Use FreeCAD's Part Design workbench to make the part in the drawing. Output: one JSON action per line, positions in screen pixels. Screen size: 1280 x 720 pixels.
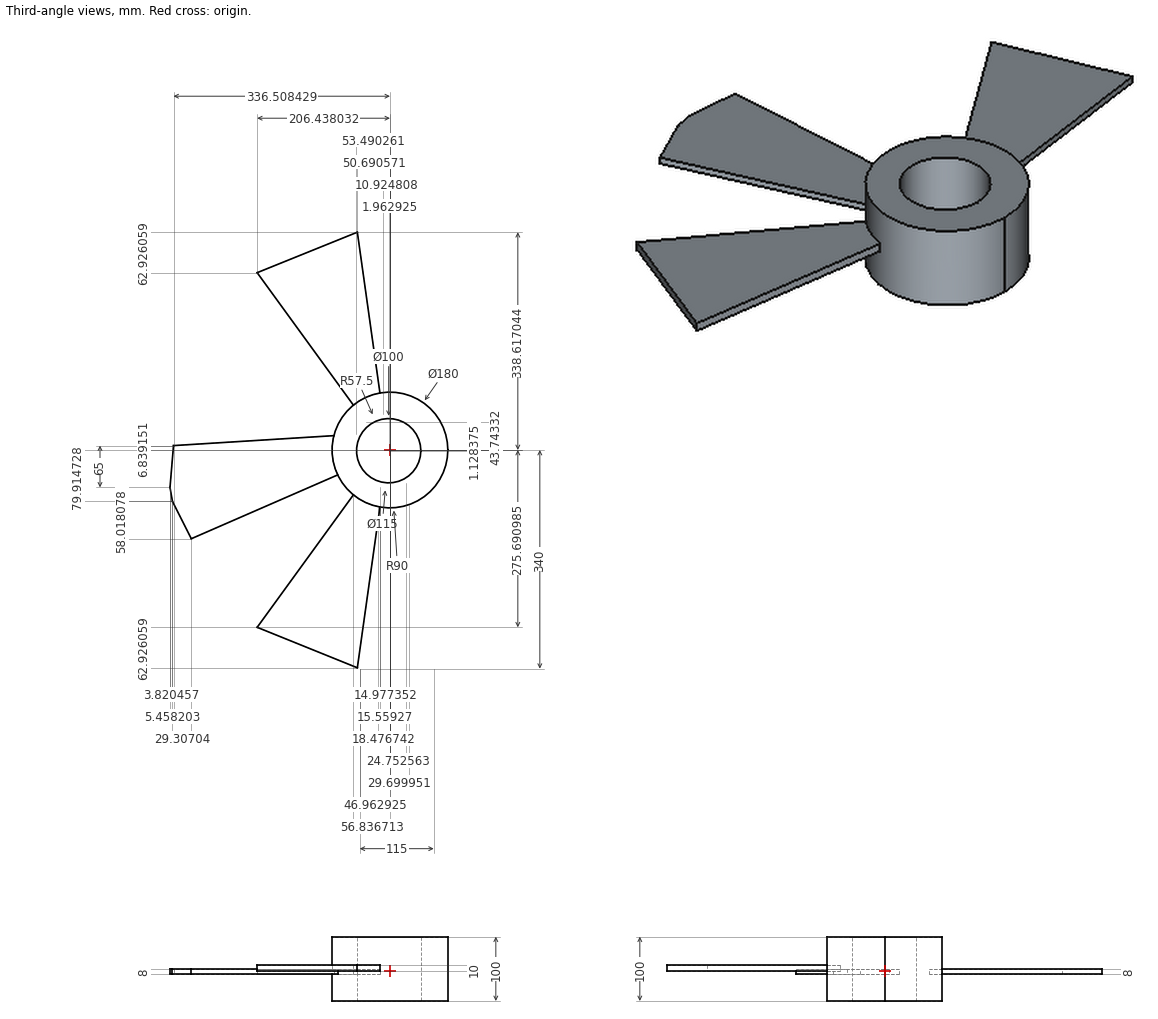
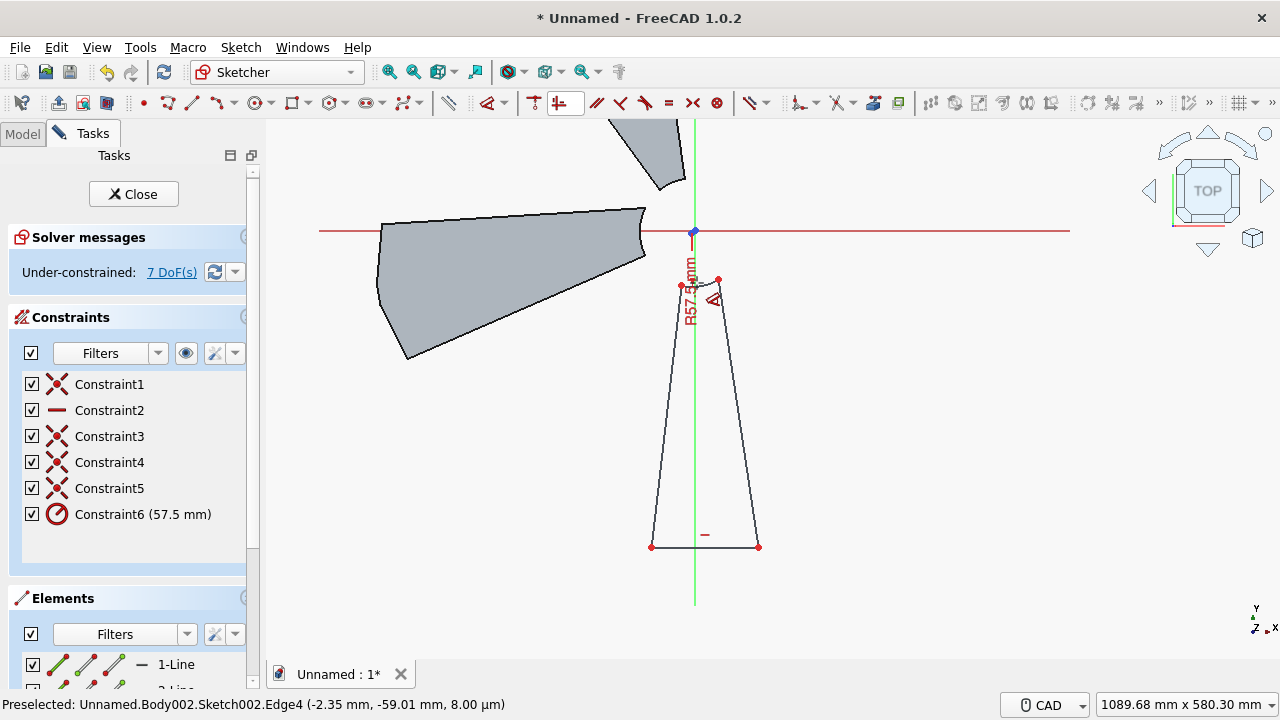
{"action": "left_click", "coordinate": [684, 548]}
{"action": "left_click", "coordinate": [680, 582]}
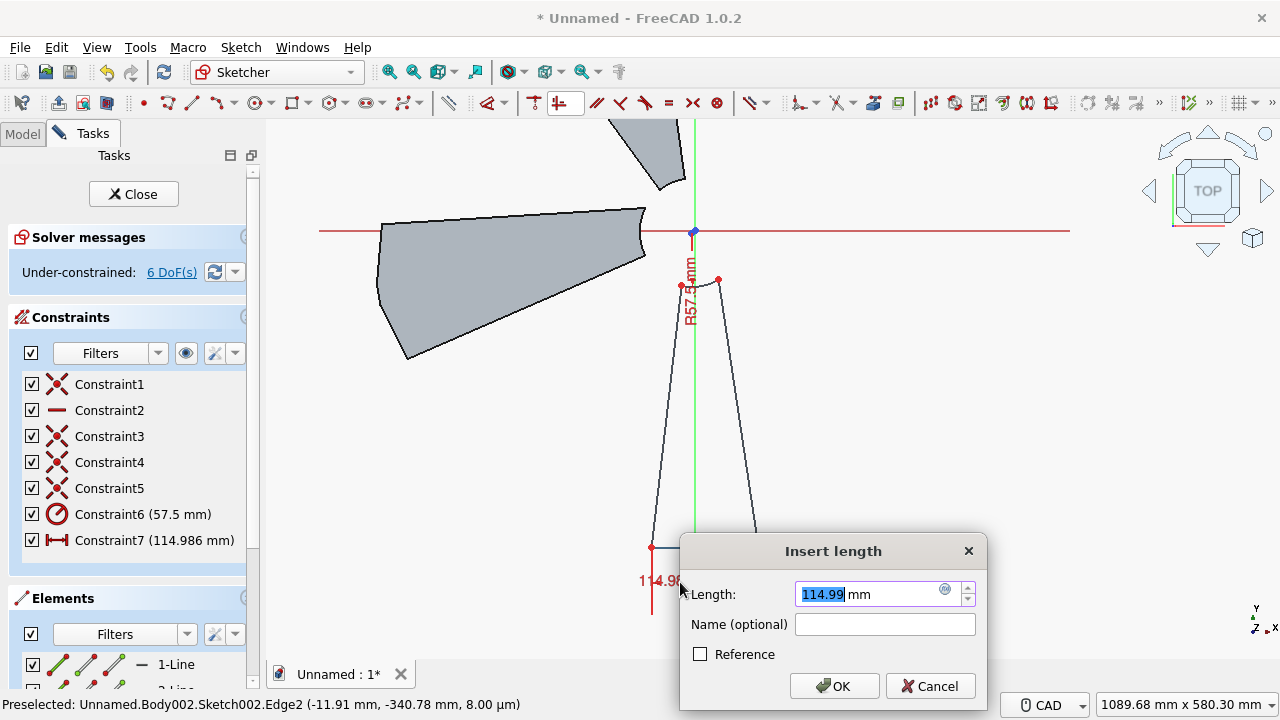
{"action": "type", "text": "115"}
{"action": "key", "text": "Return"}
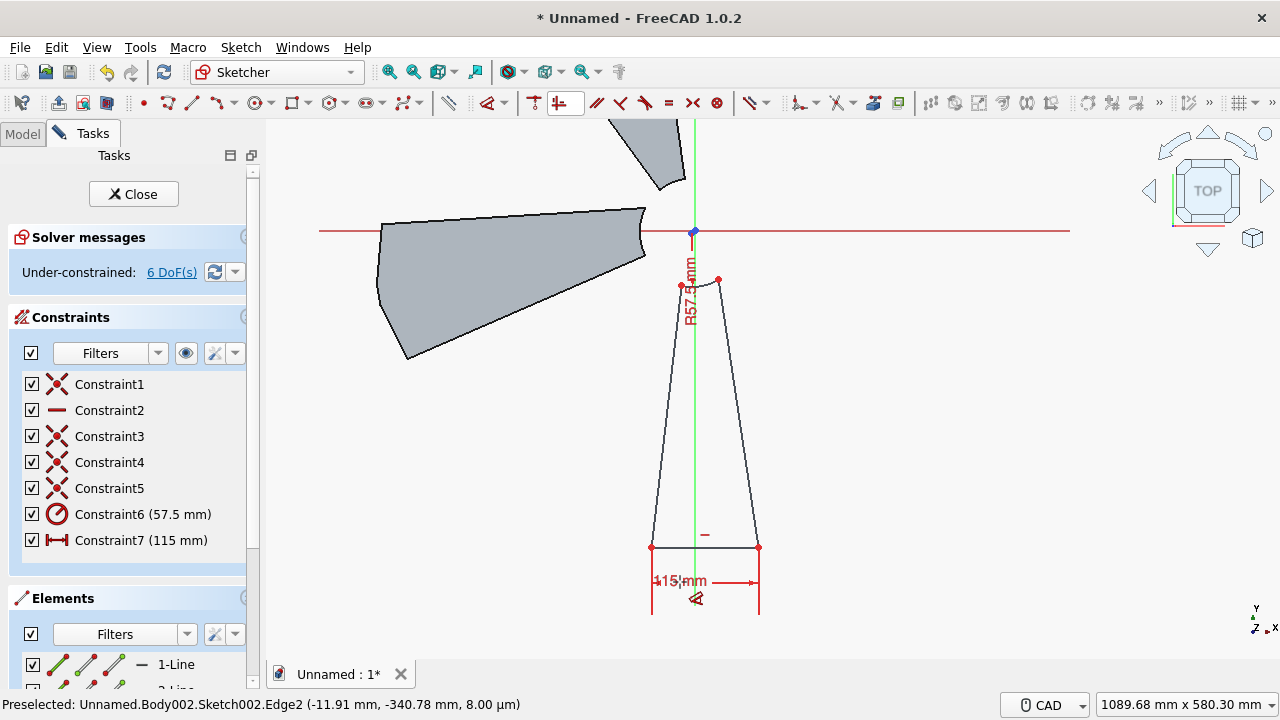
{"action": "left_click", "coordinate": [652, 548]}
{"action": "left_click", "coordinate": [618, 389]}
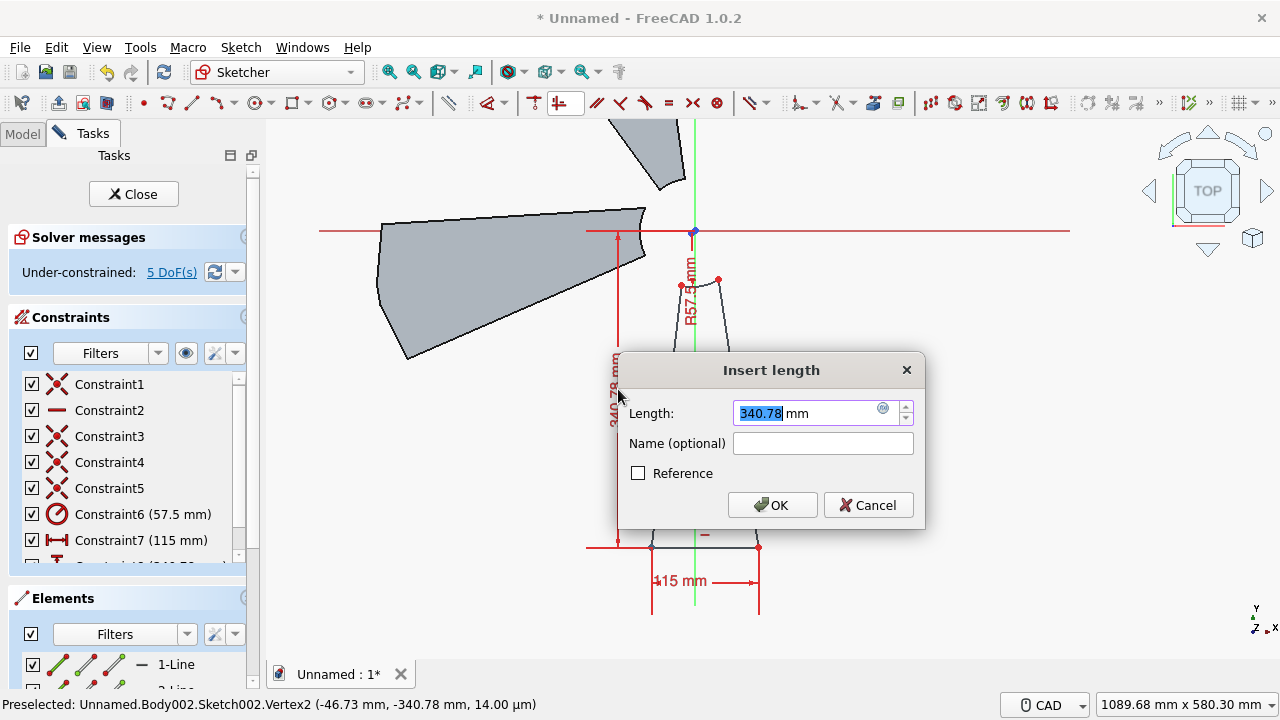
{"action": "type", "text": "340"}
{"action": "key", "text": "Return"}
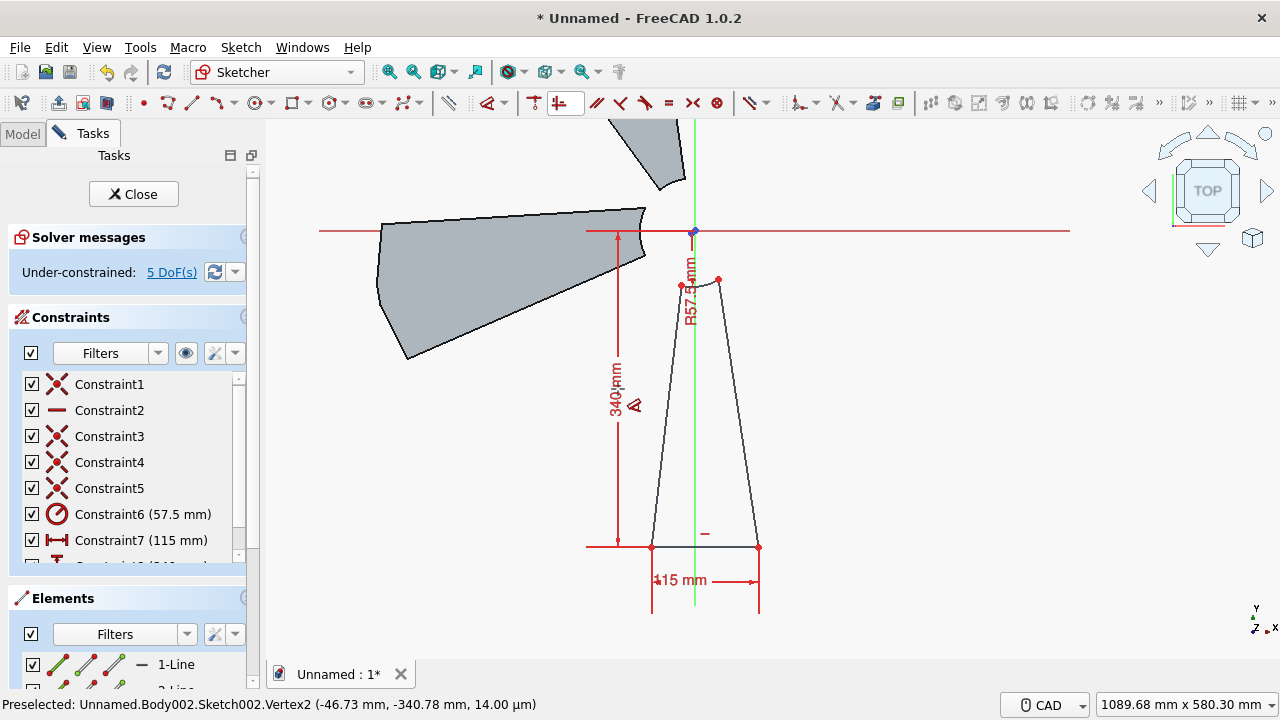
{"action": "scroll", "coordinate": [692, 233], "scroll_direction": "up", "scroll_amount": 16}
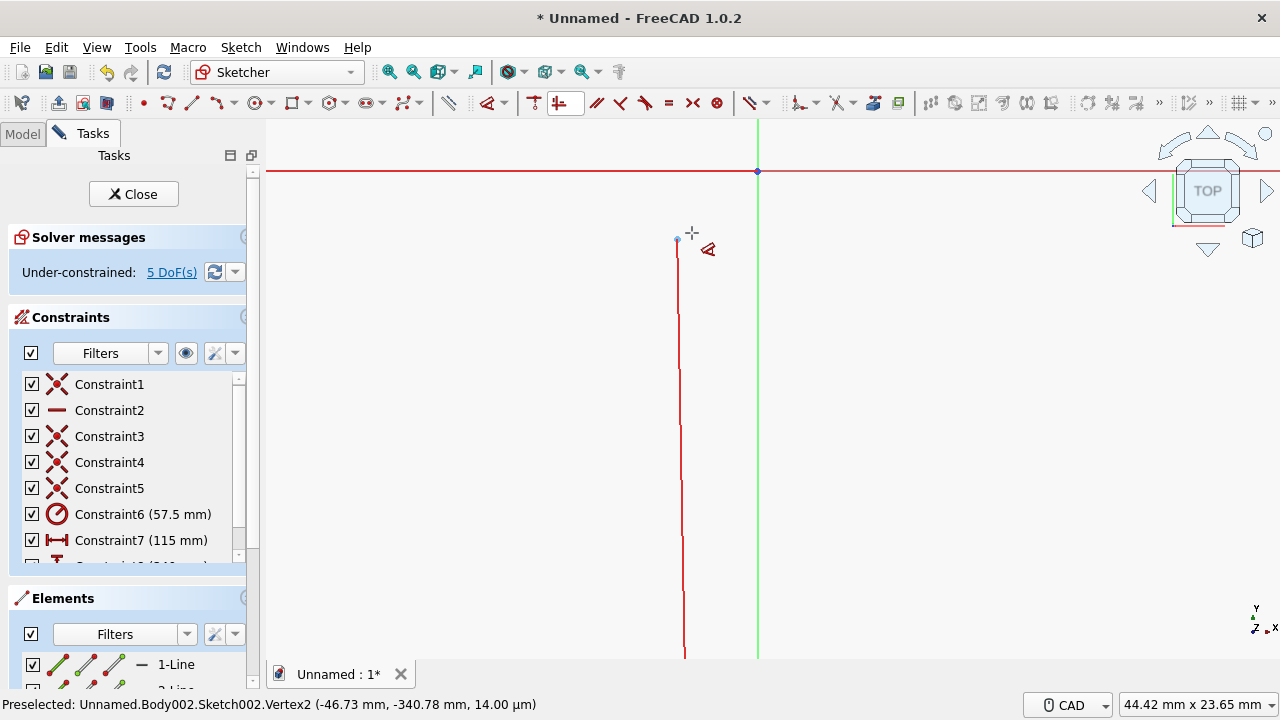
{"action": "left_click", "coordinate": [677, 239]}
{"action": "left_click", "coordinate": [717, 273]}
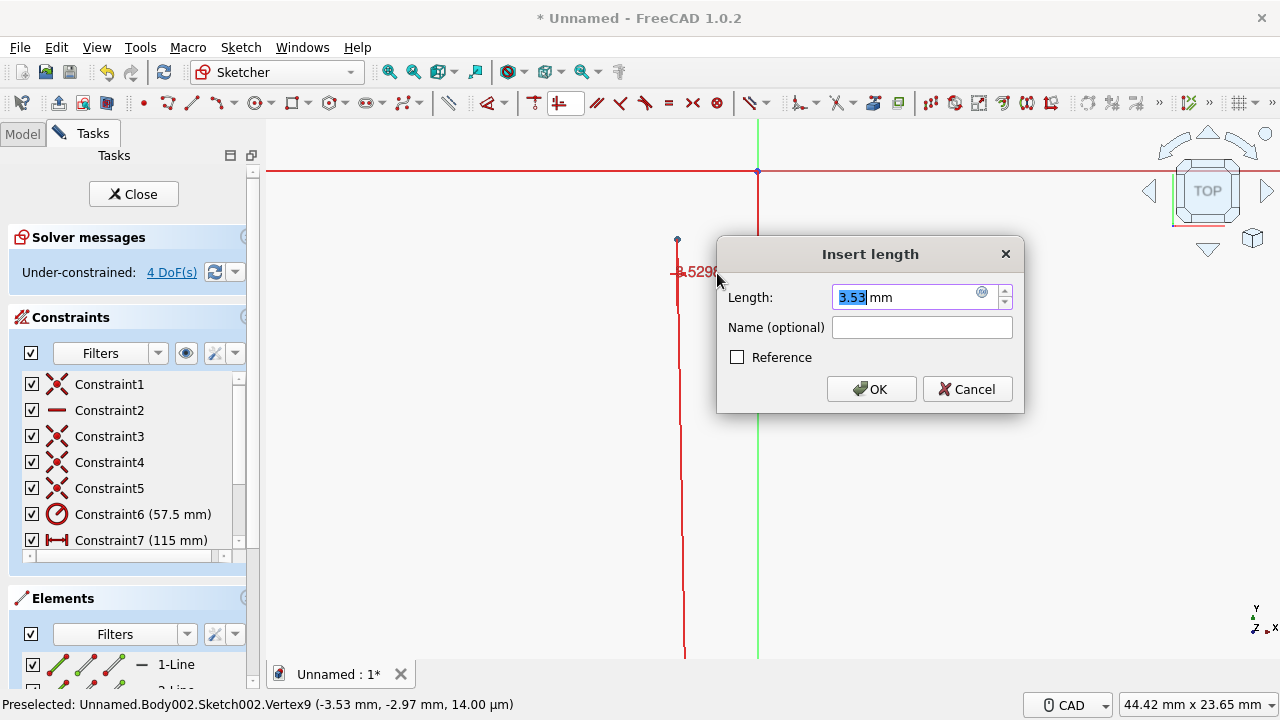
{"action": "type", "text": "1.962925"}
{"action": "key", "text": "Return"}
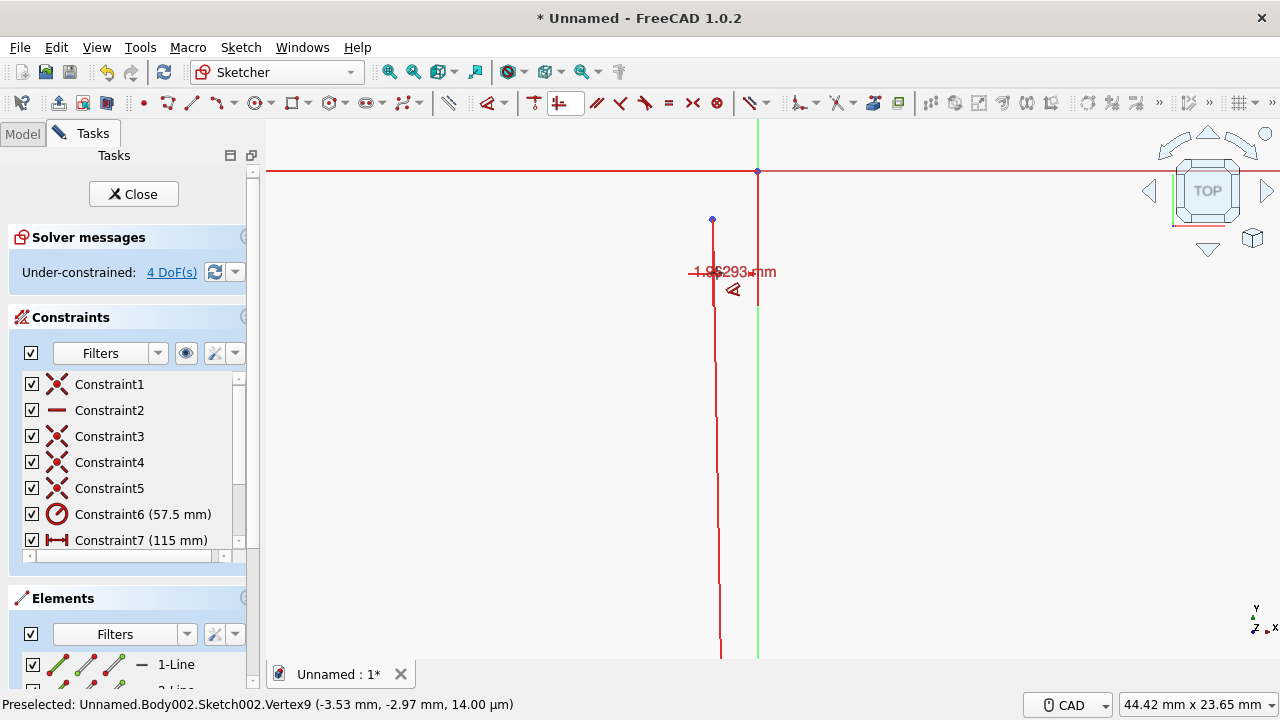
{"action": "scroll", "coordinate": [713, 219], "scroll_direction": "up", "scroll_amount": 3}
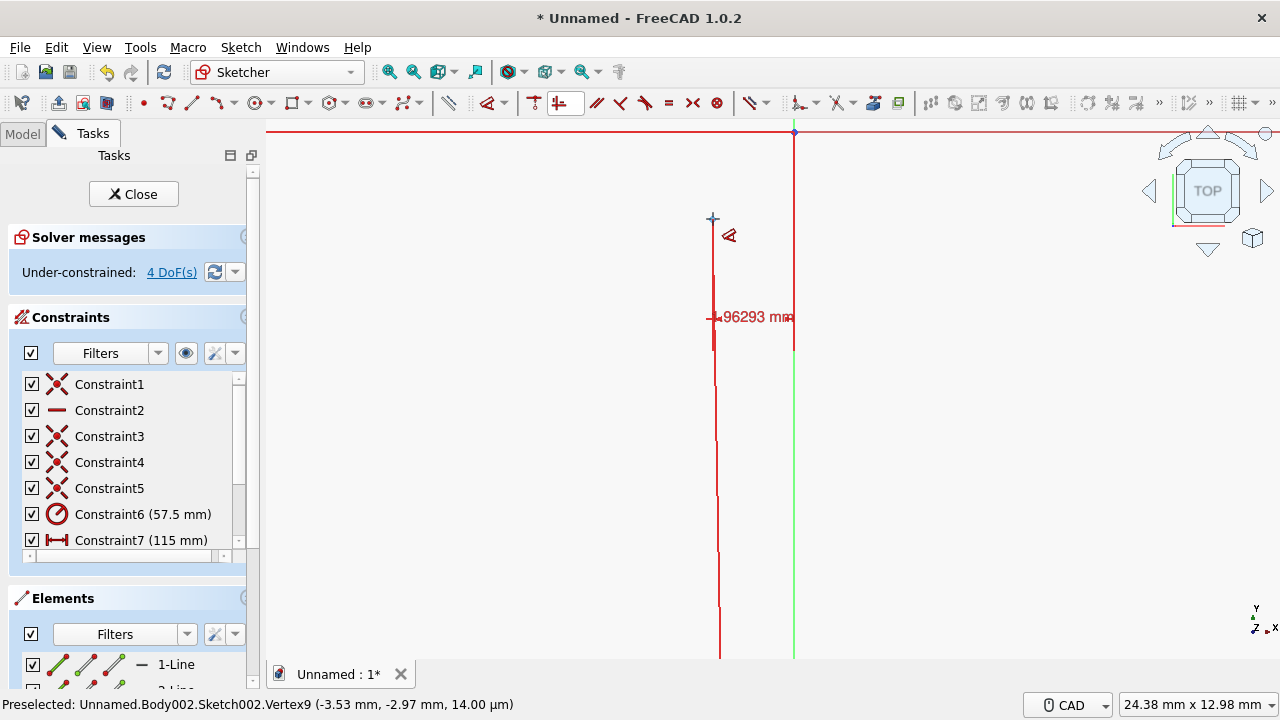
{"action": "left_click", "coordinate": [713, 219]}
{"action": "left_click", "coordinate": [679, 183]}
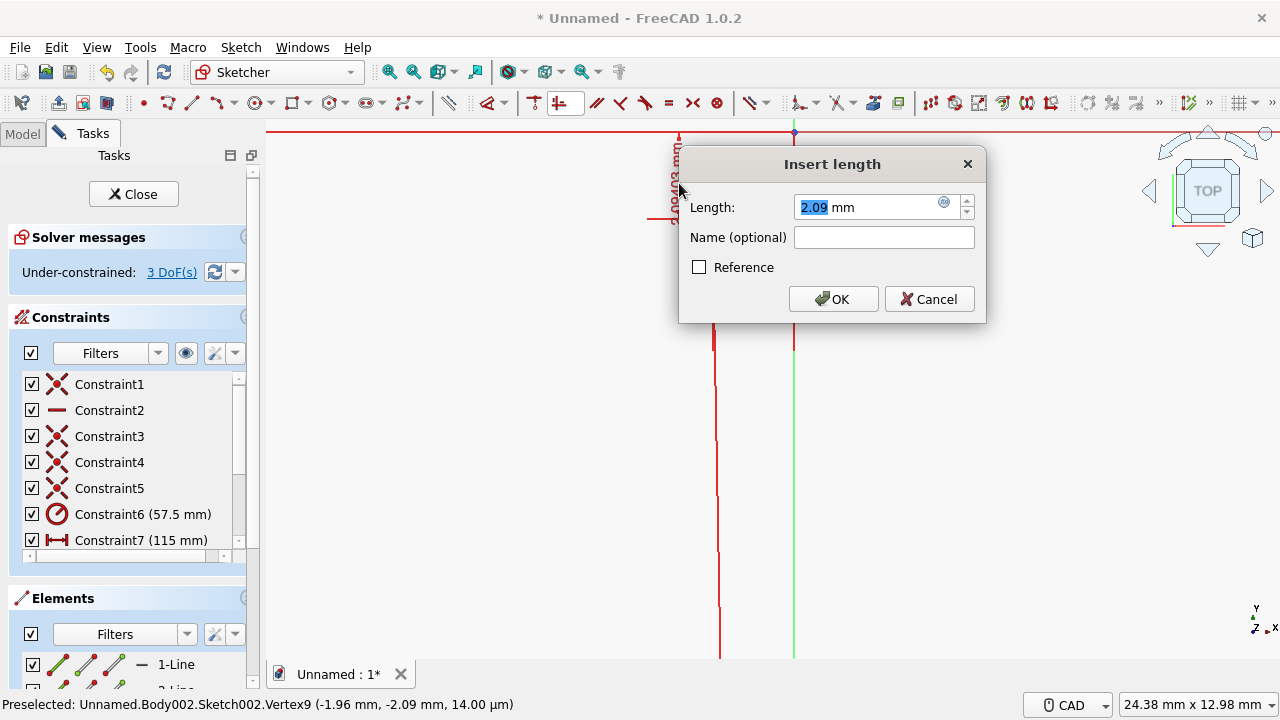
{"action": "type", "text": "1.128375"}
{"action": "key", "text": "Return"}